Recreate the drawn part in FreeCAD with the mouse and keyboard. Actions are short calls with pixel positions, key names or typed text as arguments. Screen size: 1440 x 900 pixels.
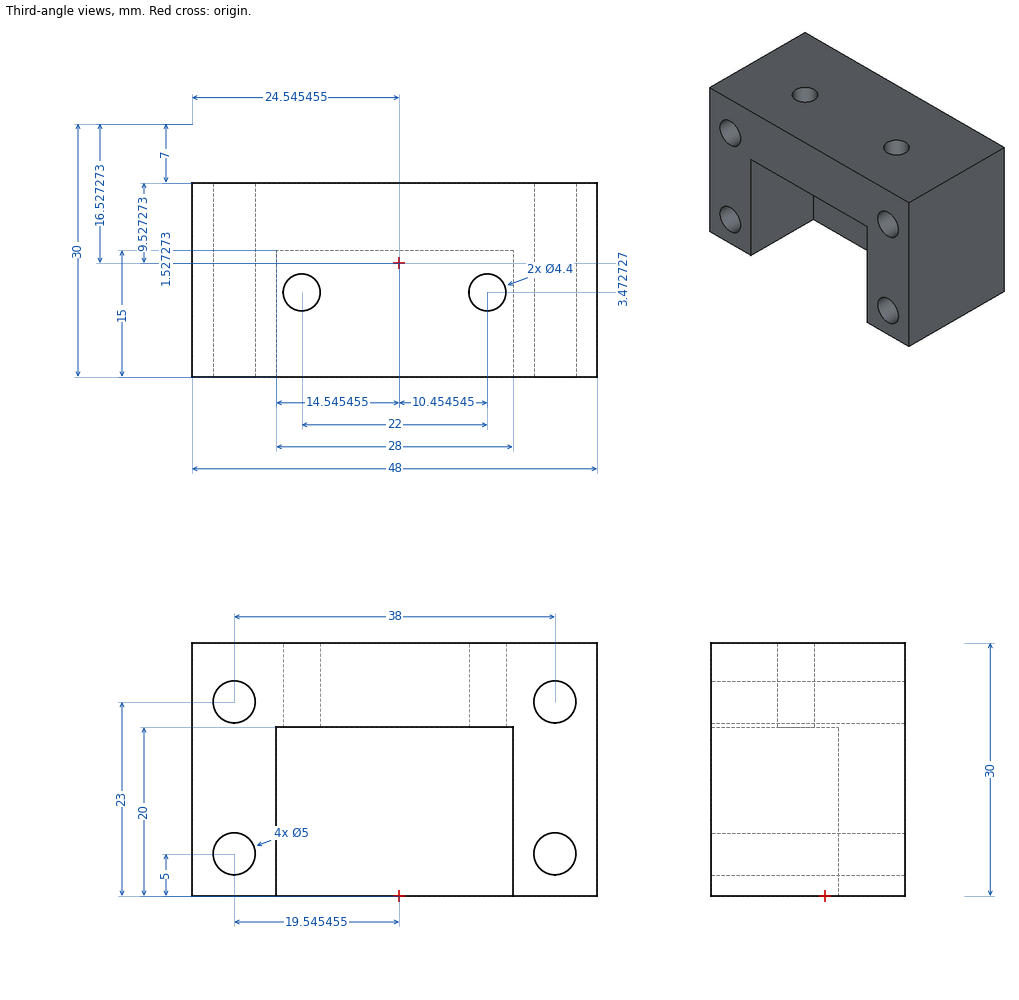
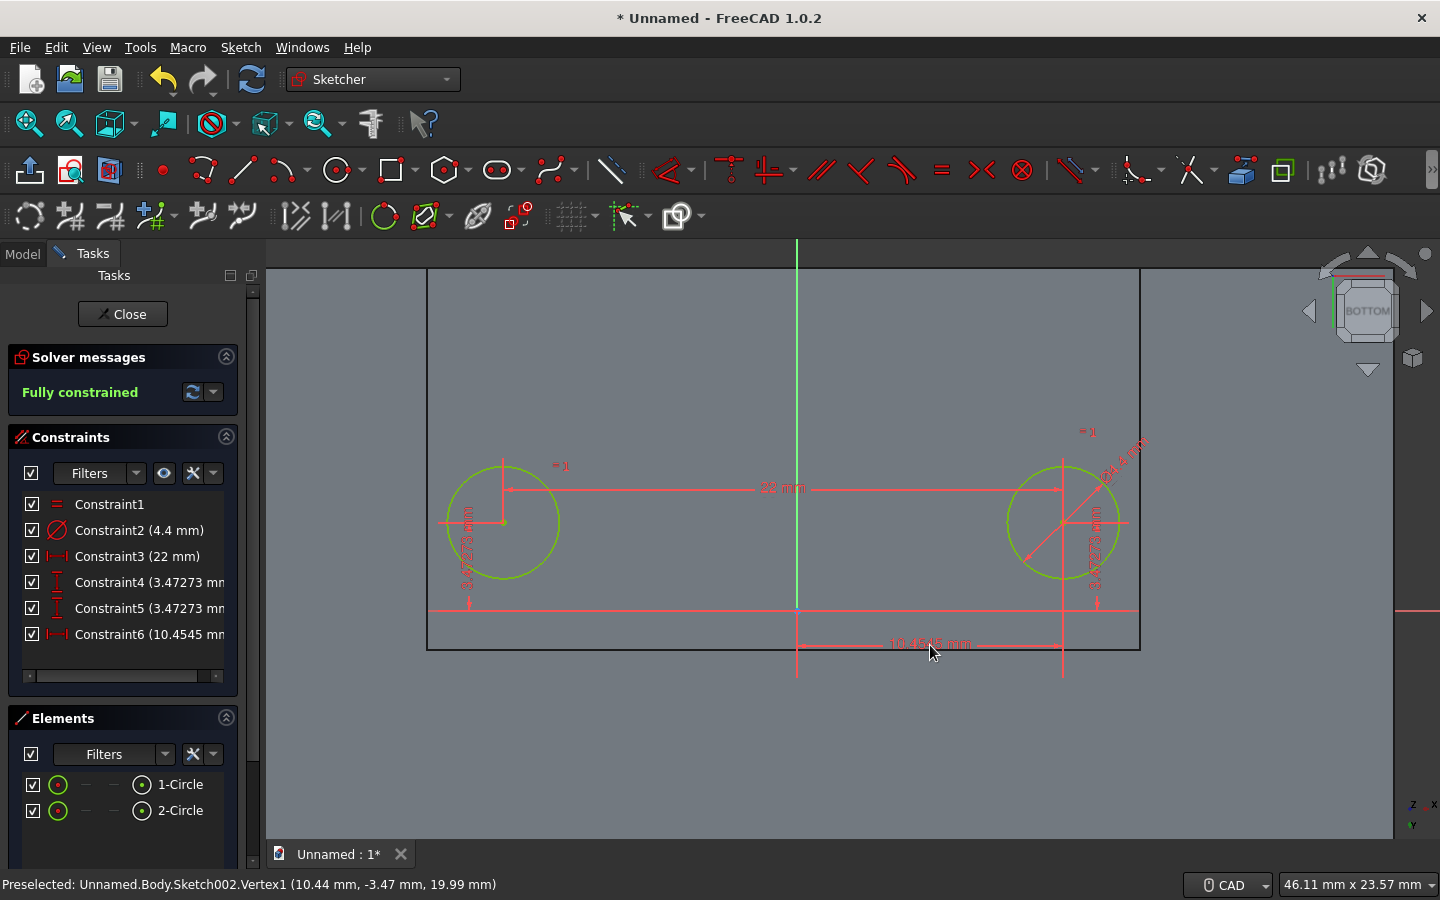
click(123, 314)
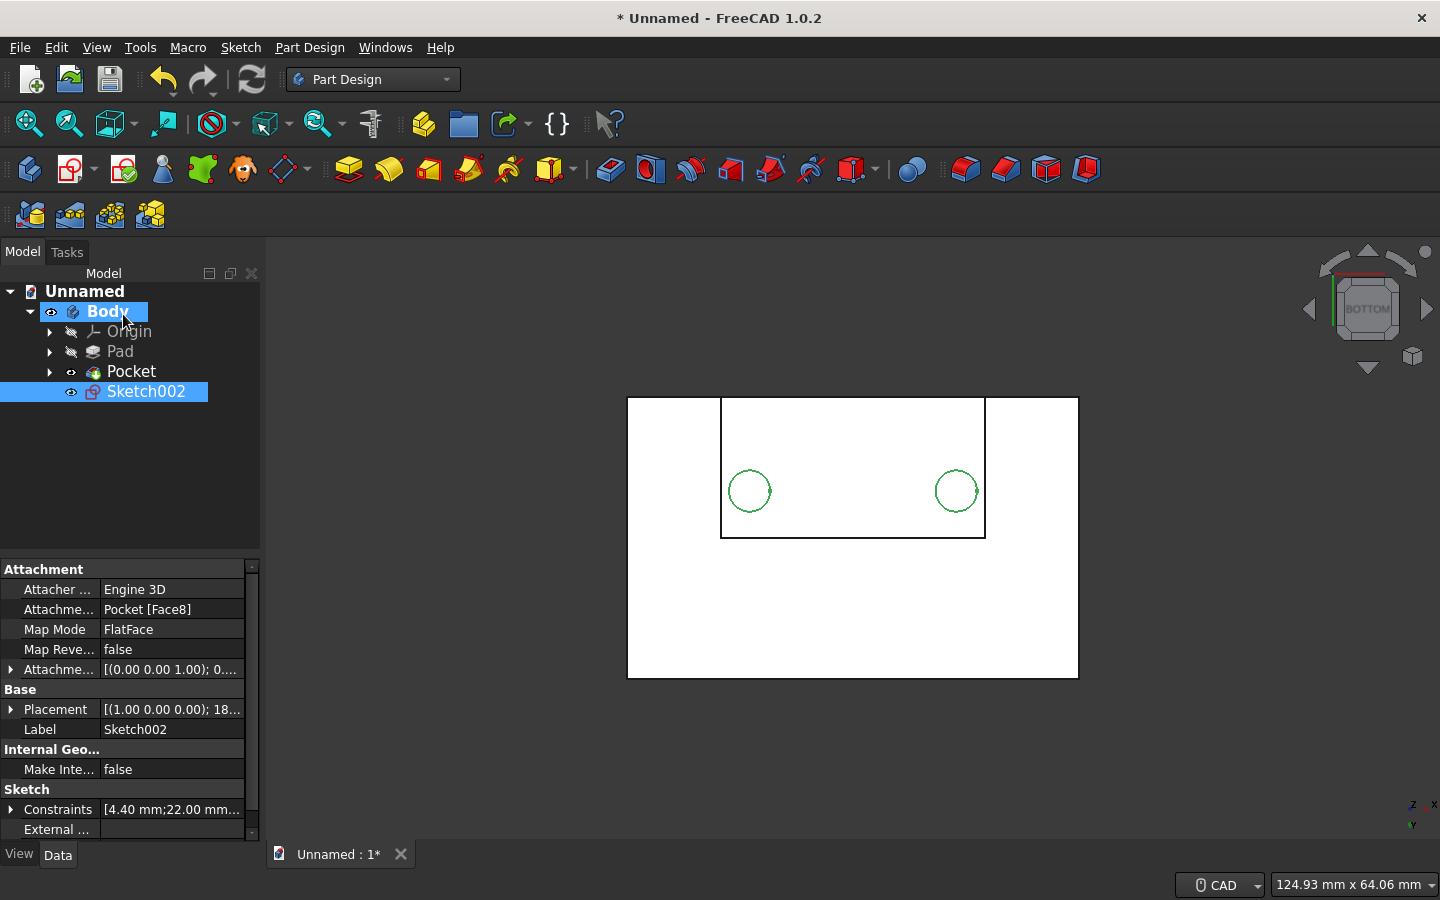
click(612, 170)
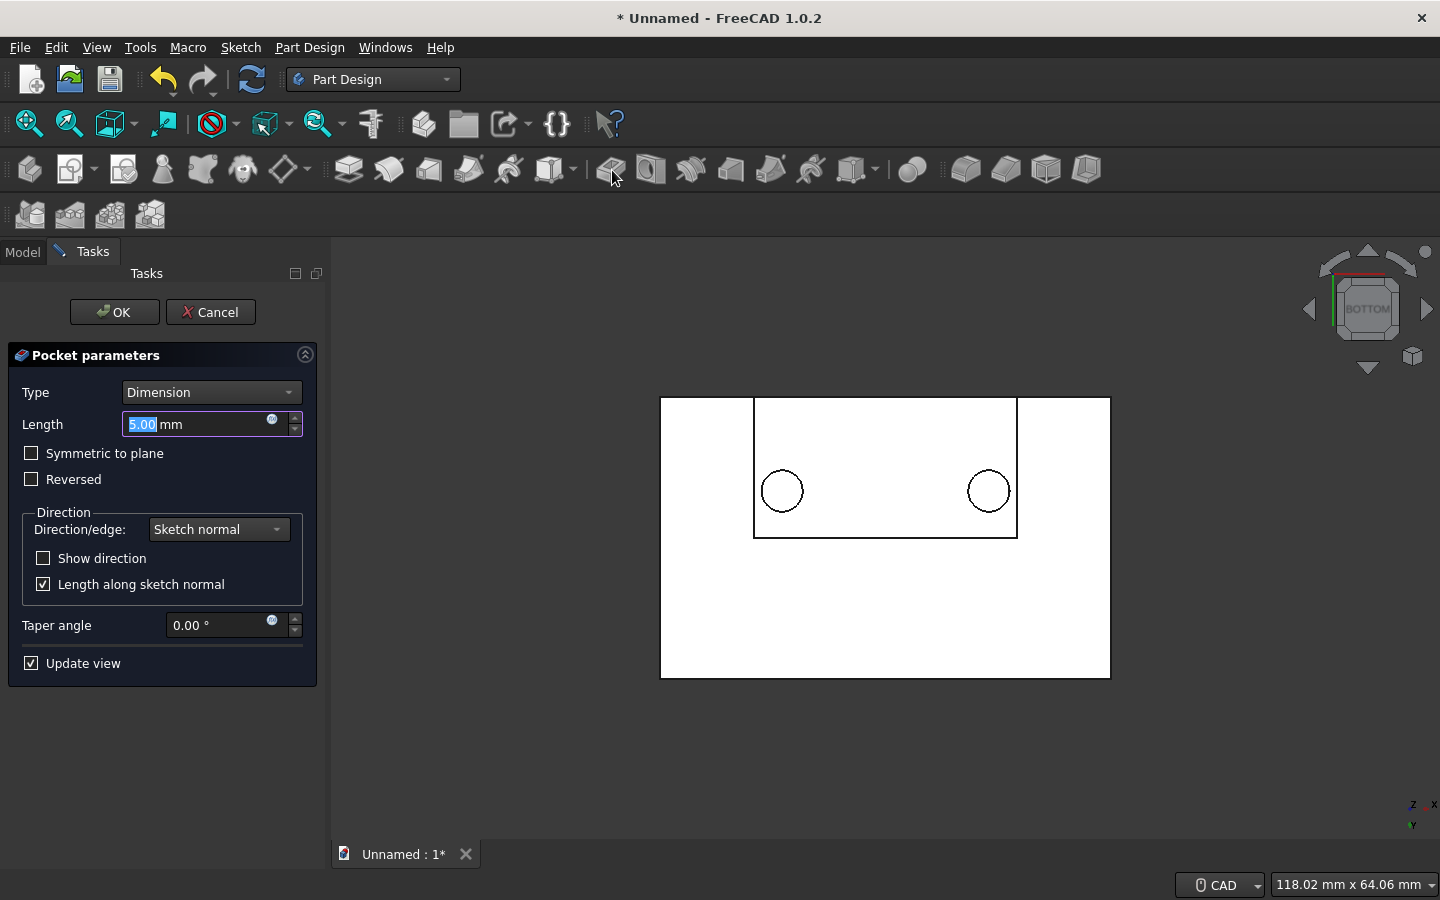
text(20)
key(Tab)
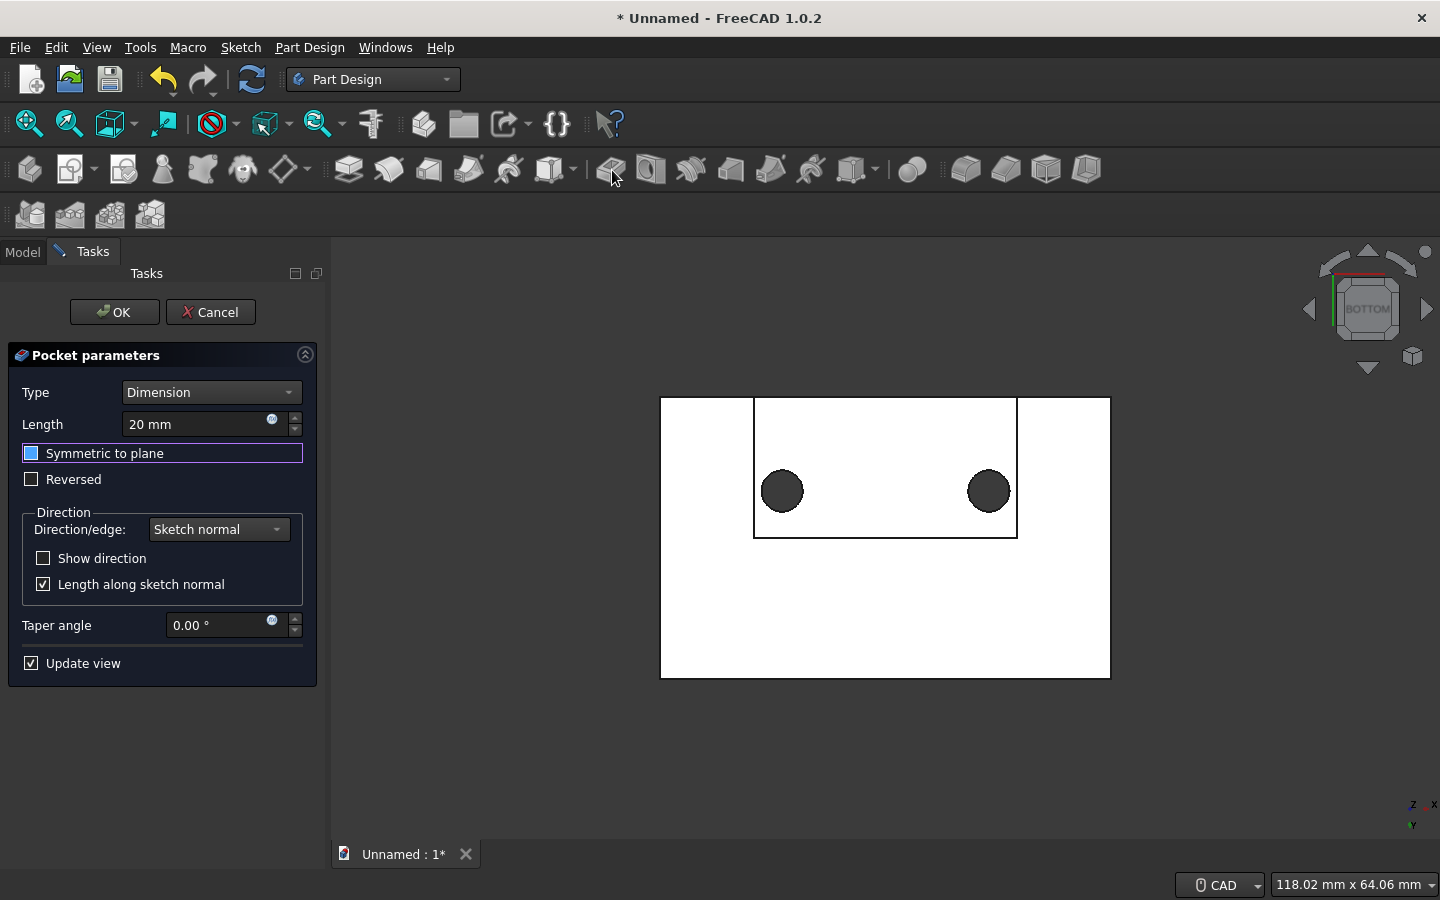
click(115, 312)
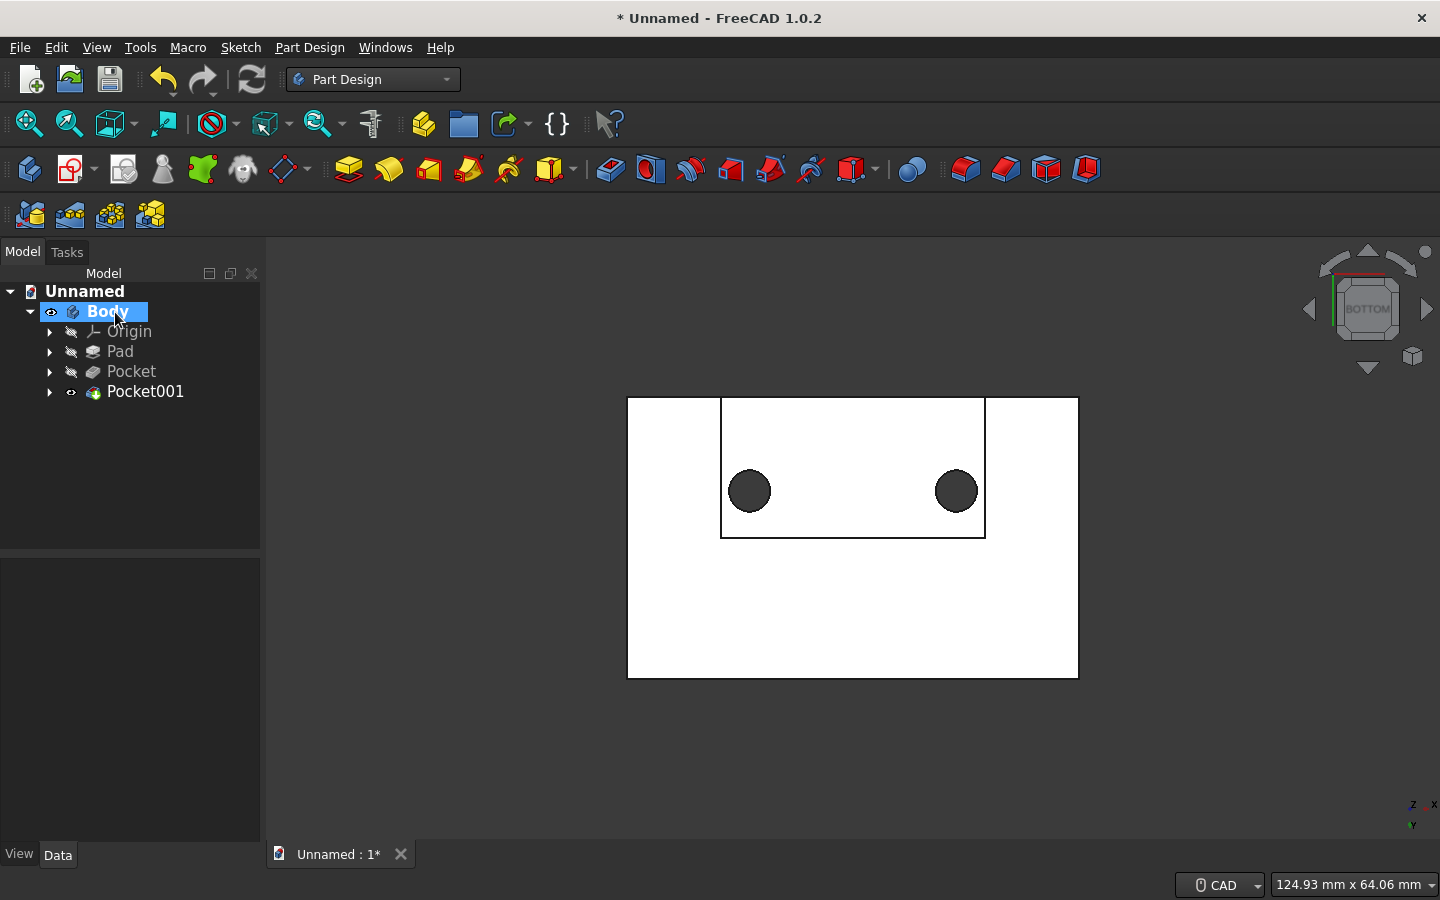
key(0)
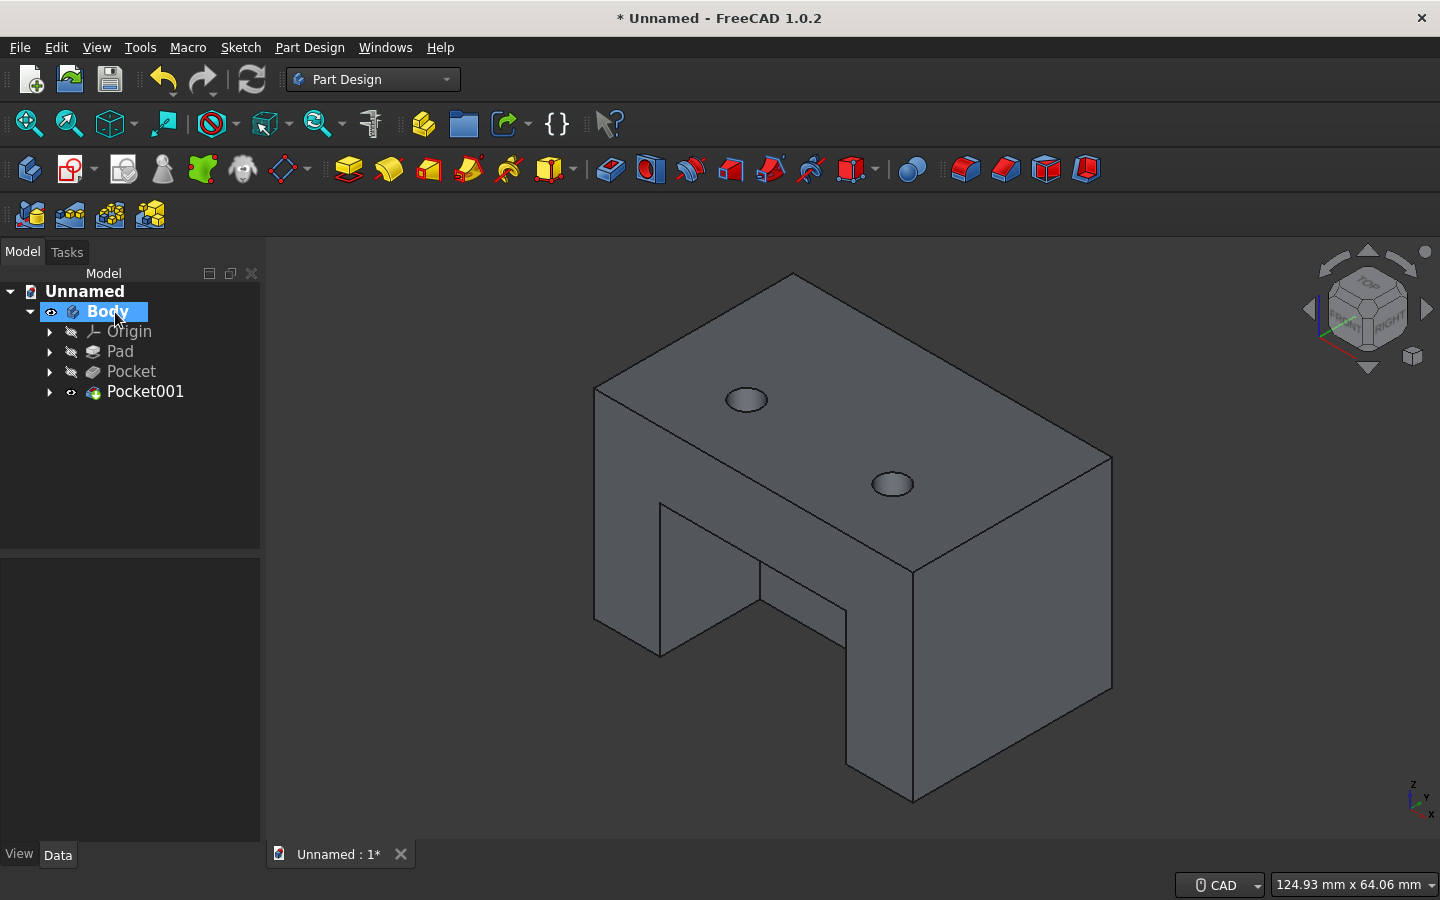
click(844, 581)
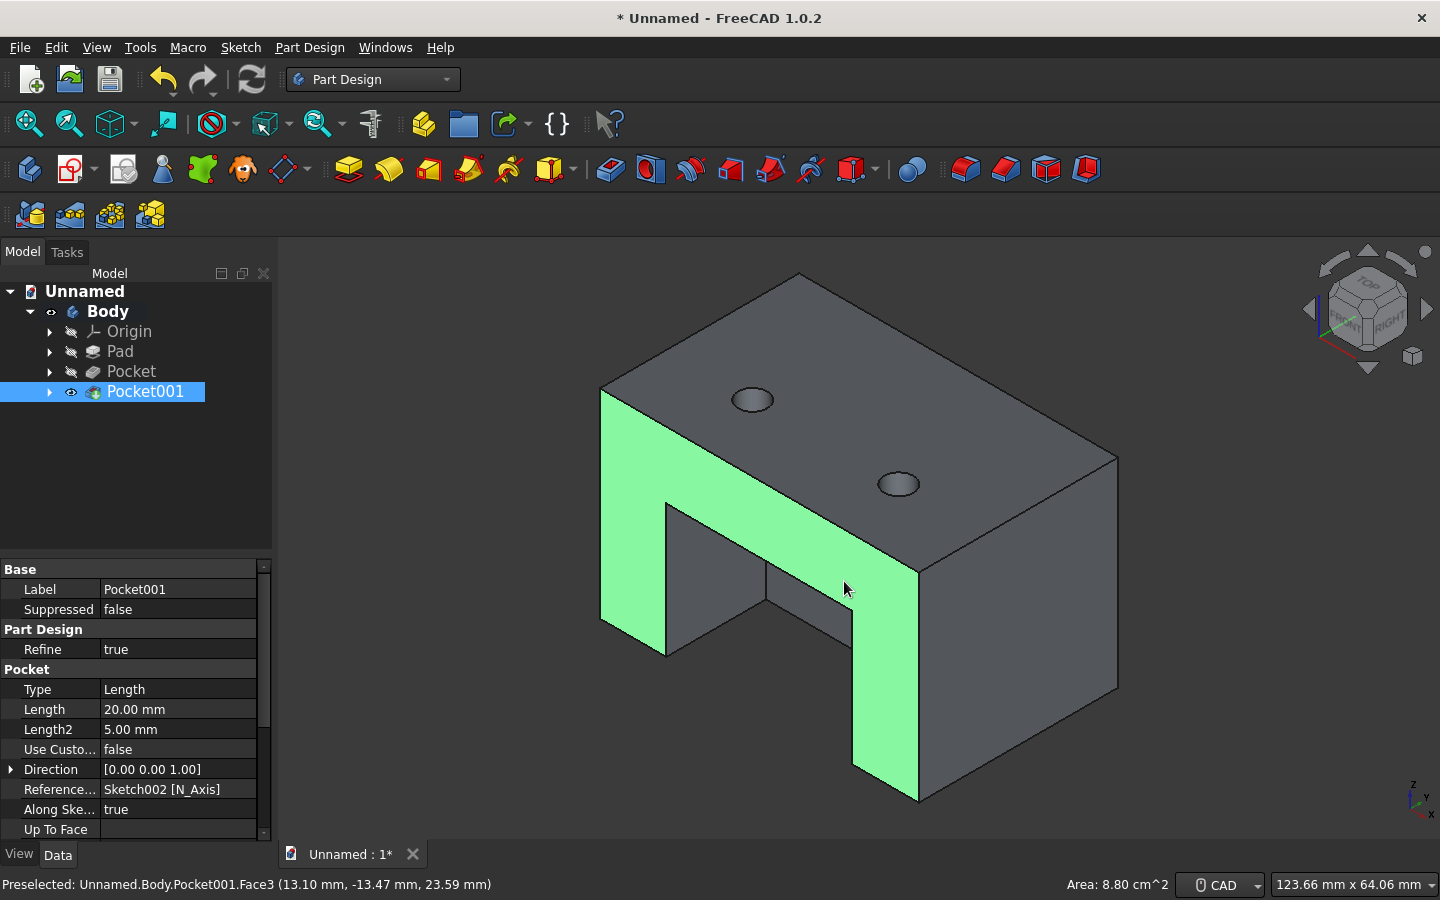
click(70, 170)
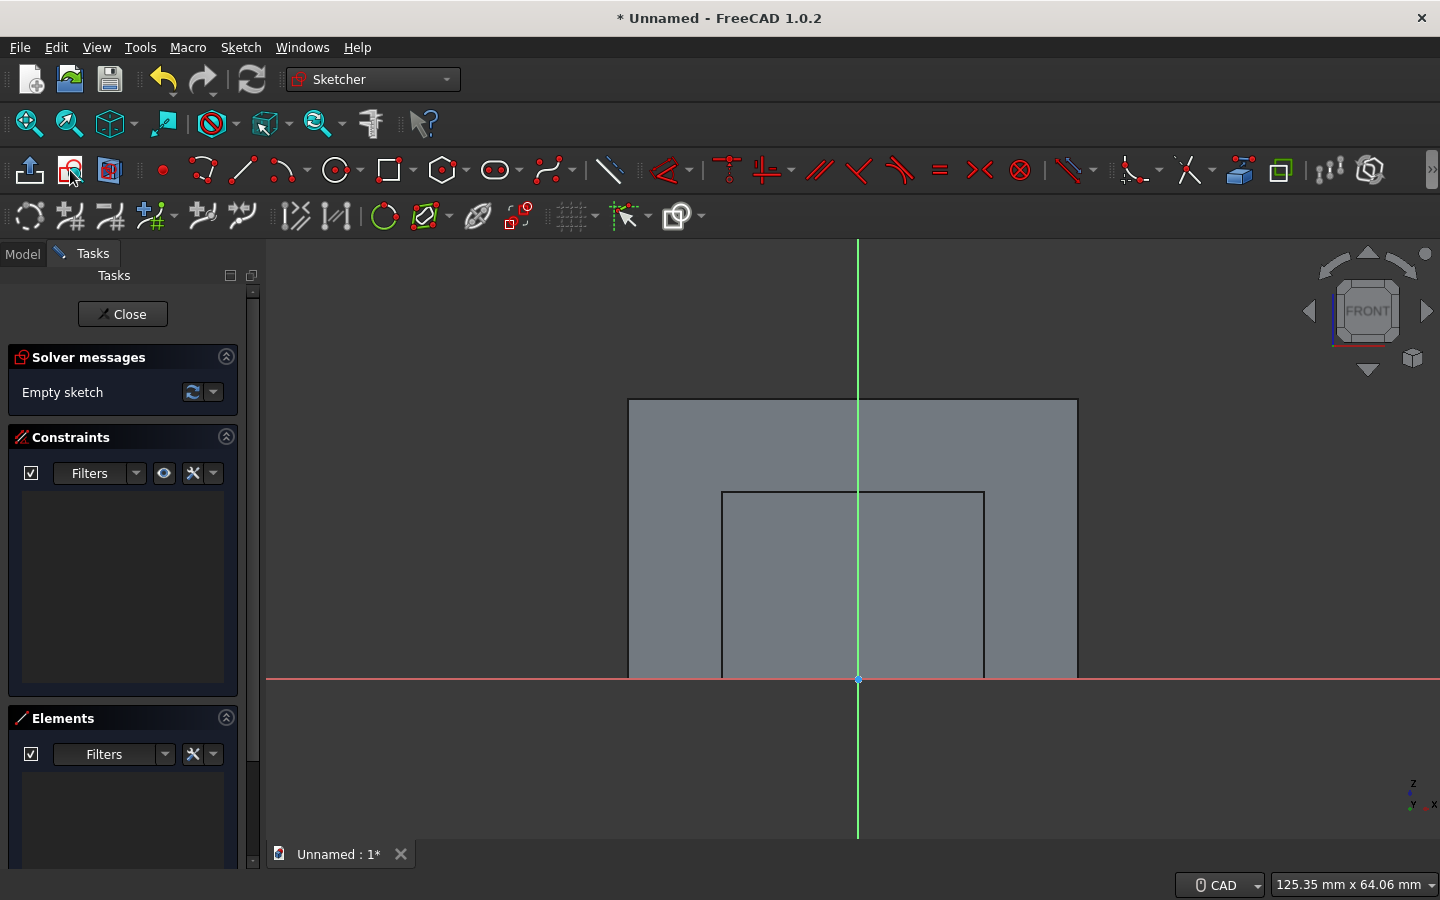
scroll(992, 603, up, 2)